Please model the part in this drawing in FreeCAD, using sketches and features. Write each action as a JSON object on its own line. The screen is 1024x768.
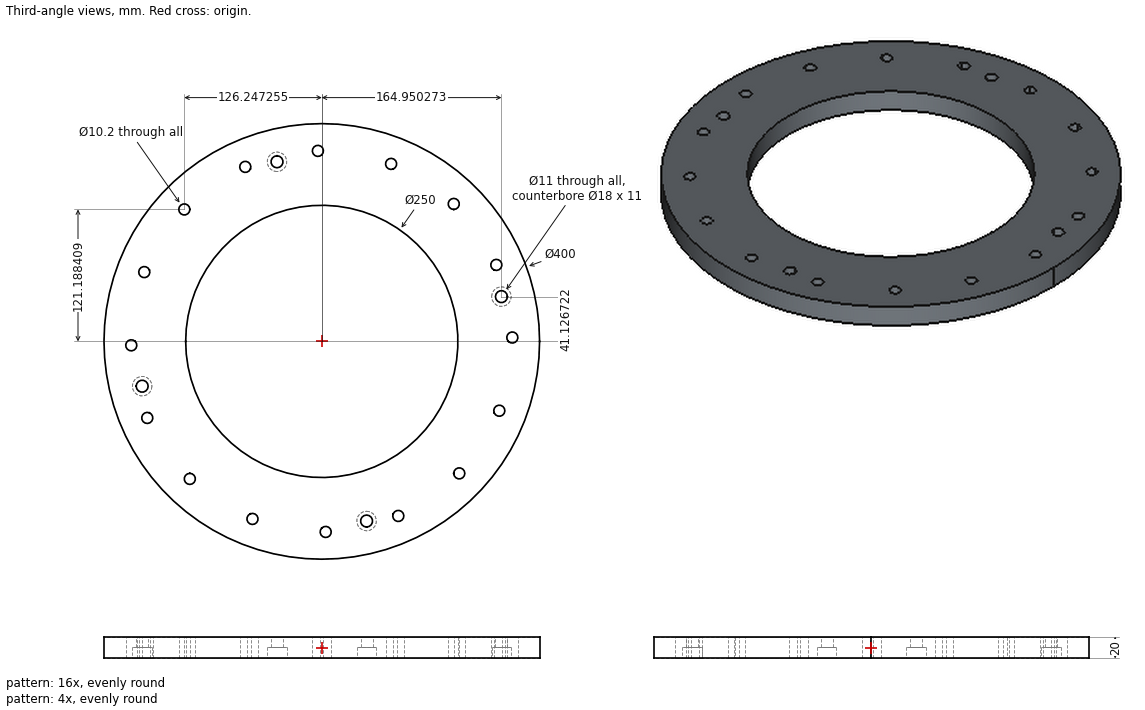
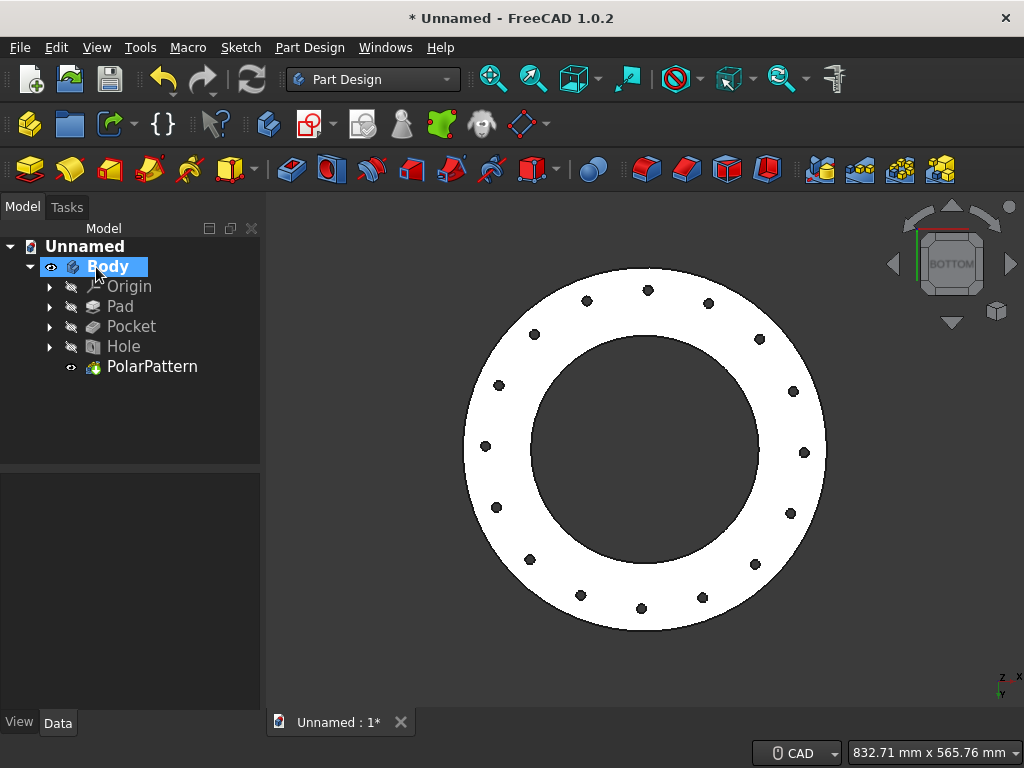
{"action": "left_click", "coordinate": [489, 396]}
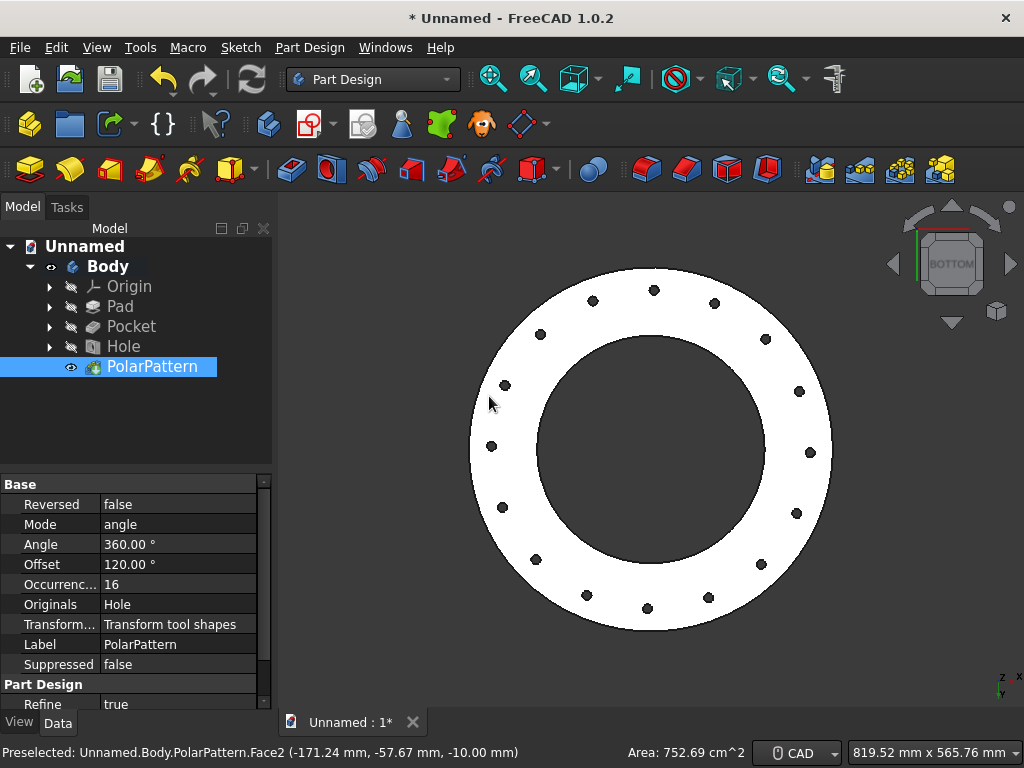
{"action": "left_click", "coordinate": [310, 124]}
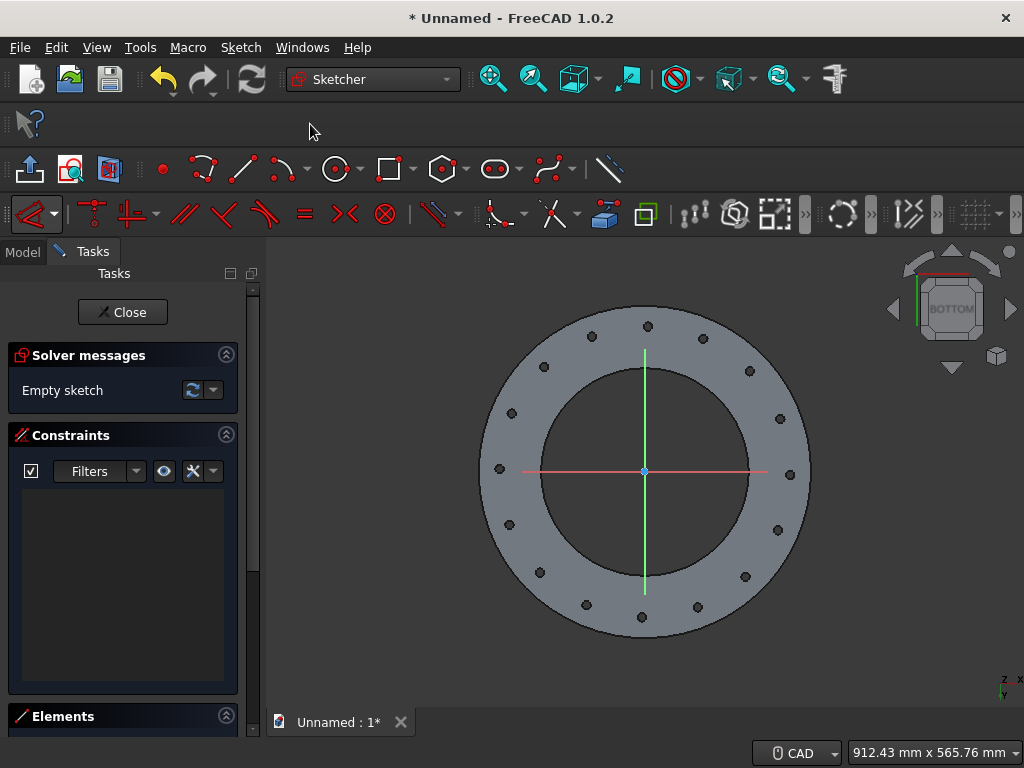
{"action": "scroll", "coordinate": [793, 508], "scroll_direction": "up", "scroll_amount": 15}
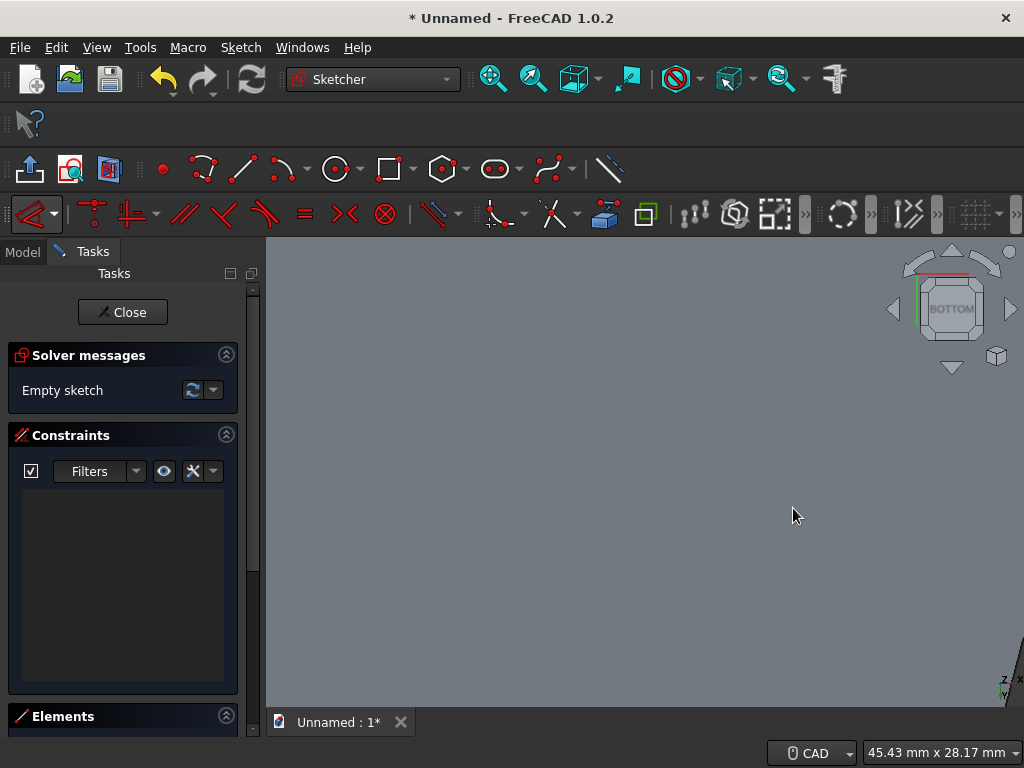
{"action": "scroll", "coordinate": [518, 436], "scroll_direction": "up", "scroll_amount": 2}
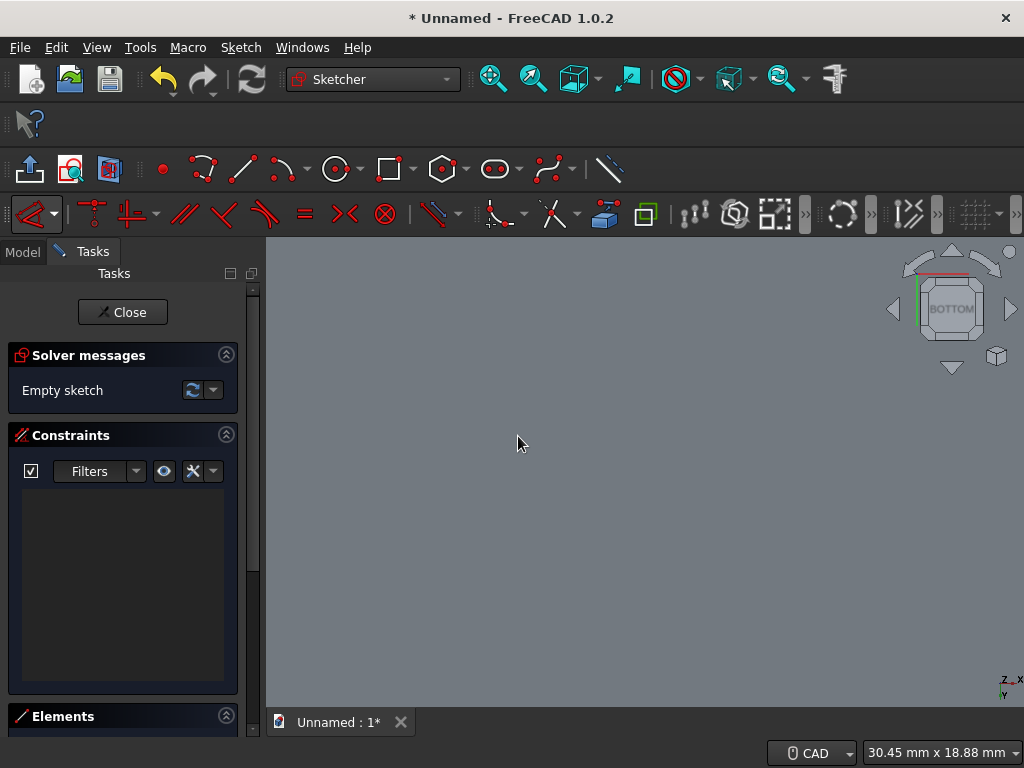
{"action": "left_click", "coordinate": [336, 170]}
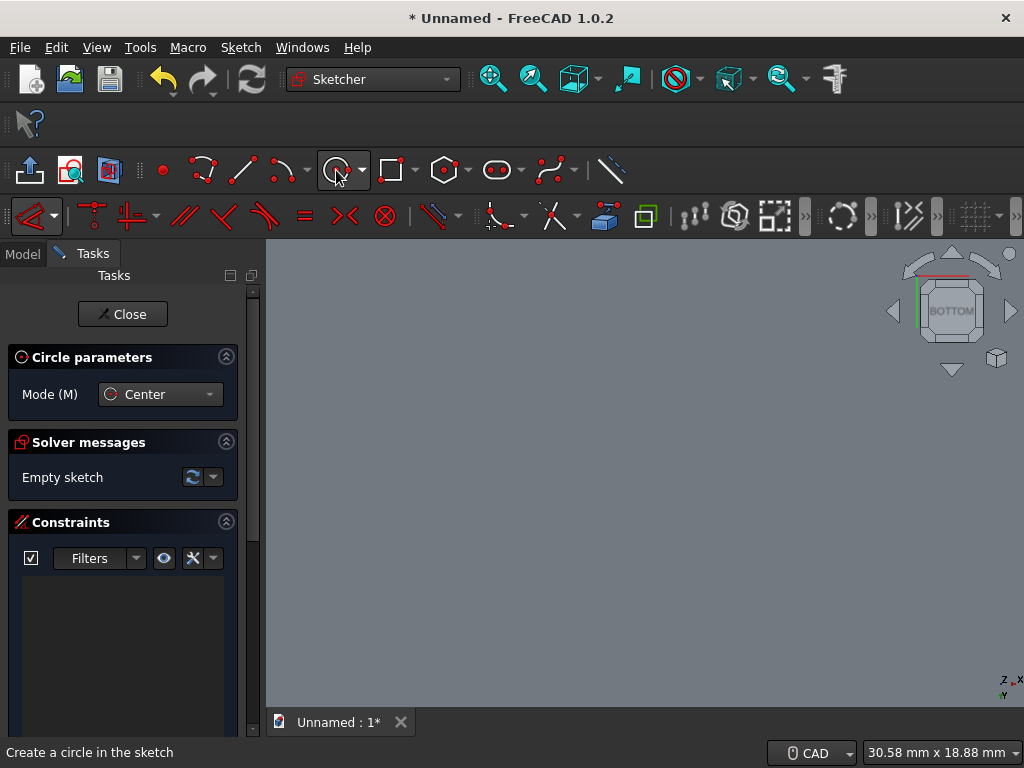
{"action": "left_click", "coordinate": [577, 473]}
{"action": "left_click", "coordinate": [673, 376]}
{"action": "key", "text": "Escape"}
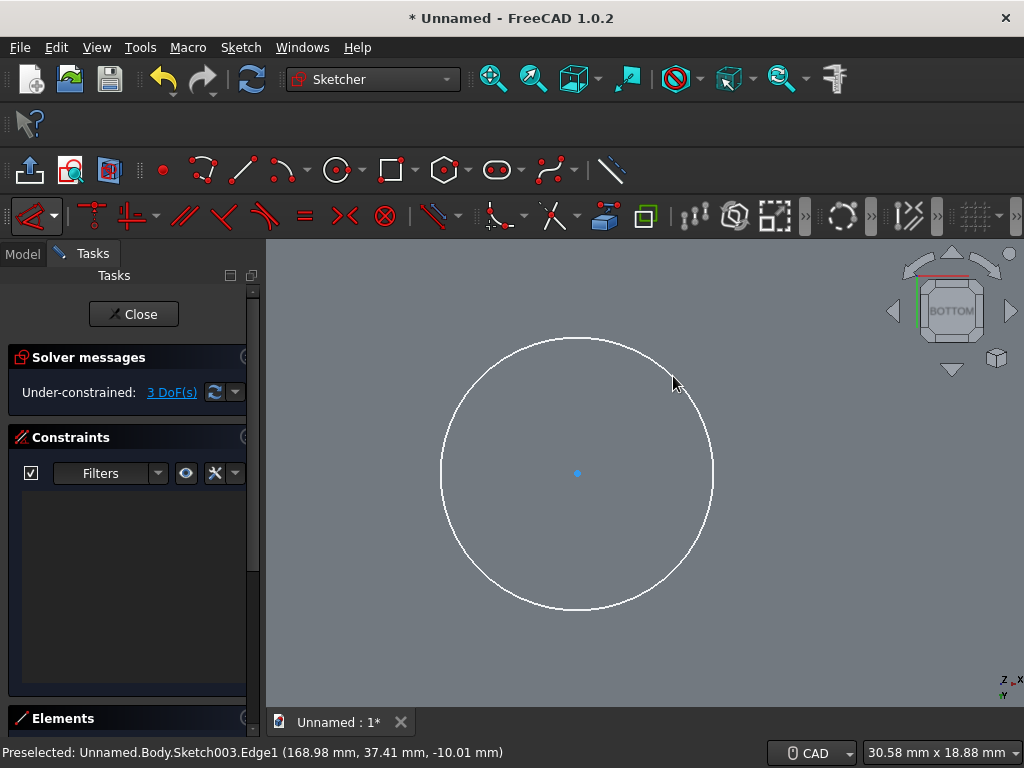
{"action": "left_click", "coordinate": [673, 377]}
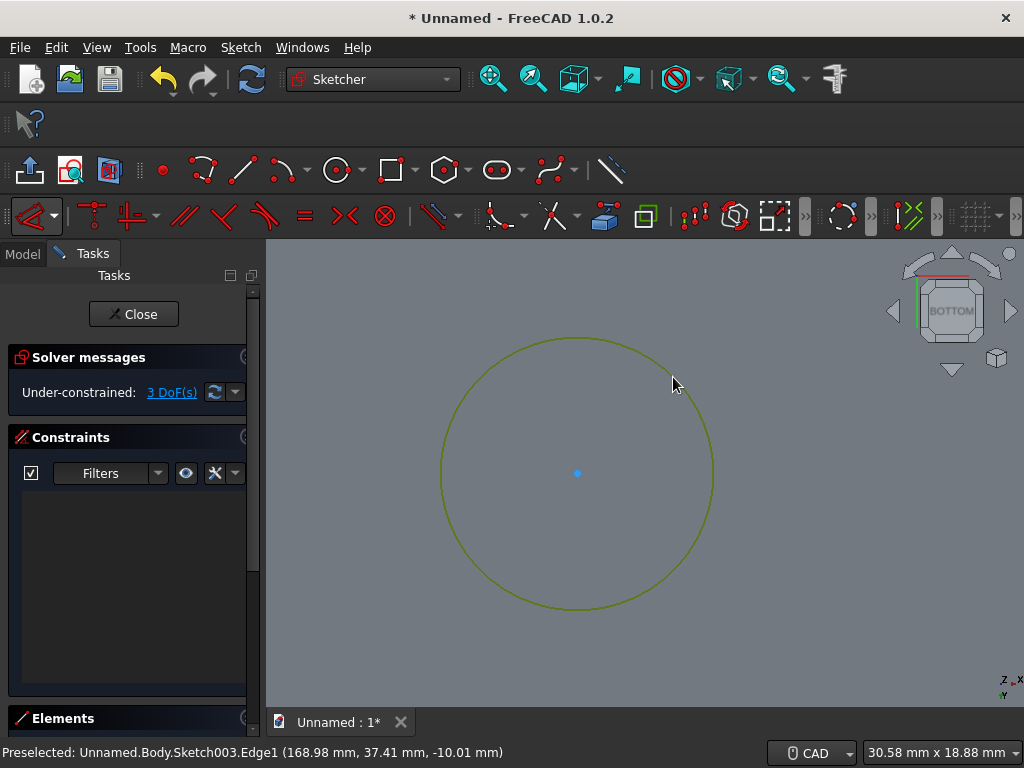
{"action": "left_click", "coordinate": [56, 216]}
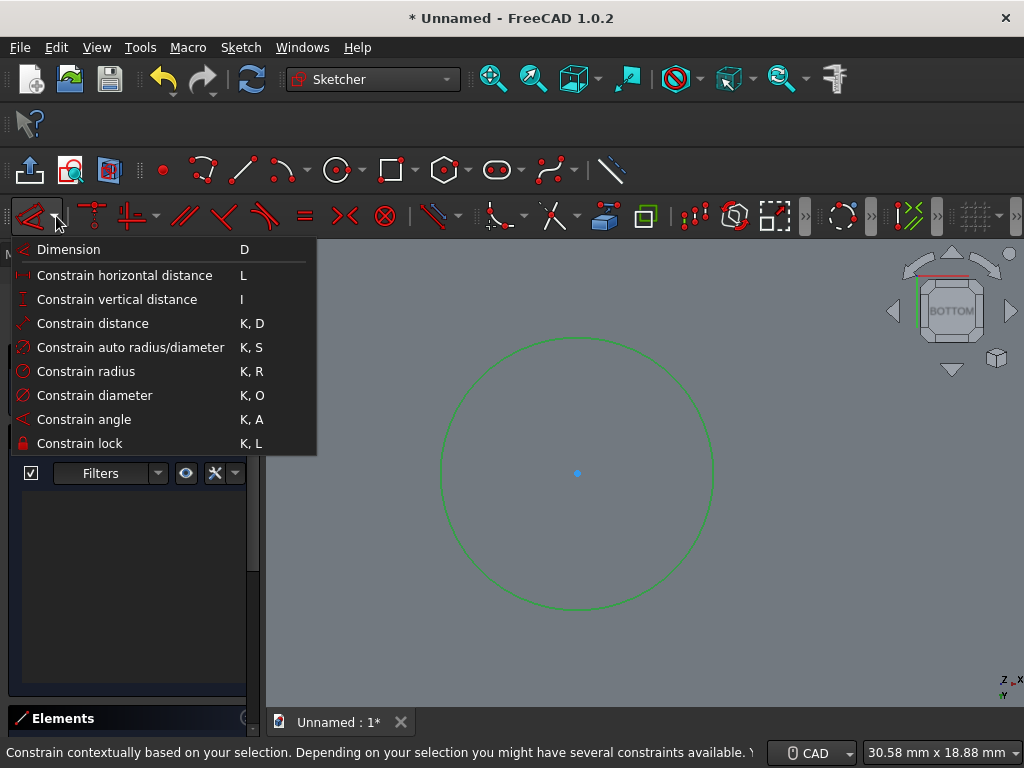
{"action": "left_click", "coordinate": [164, 395]}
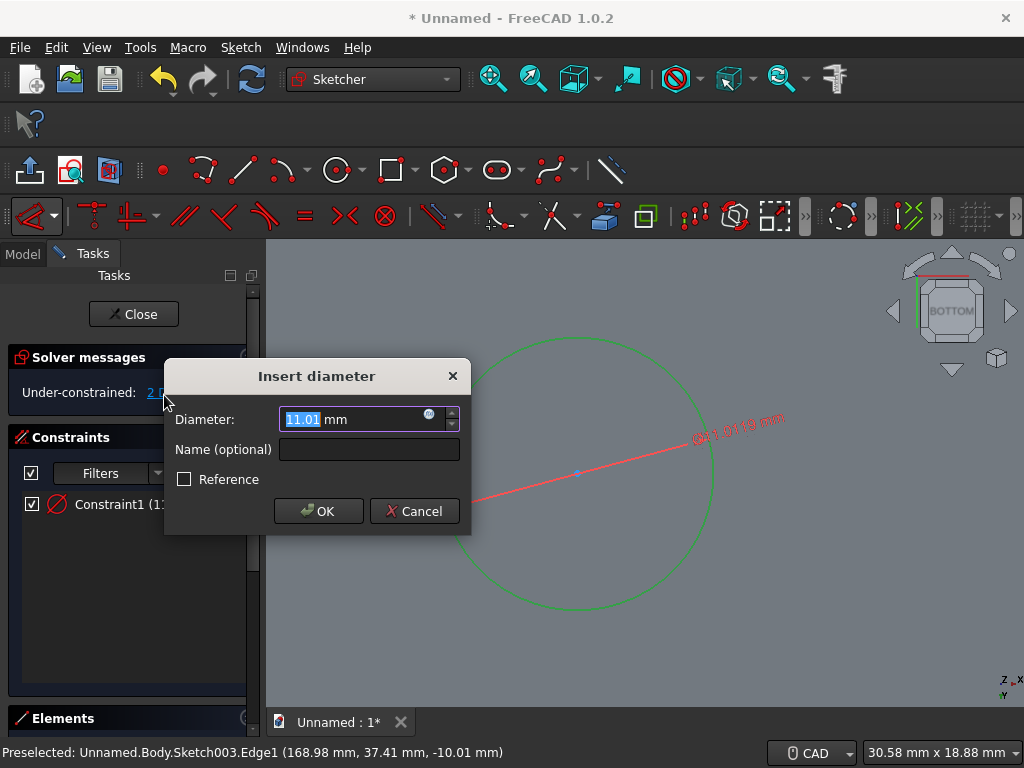
{"action": "type", "text": "11"}
{"action": "key", "text": "Return"}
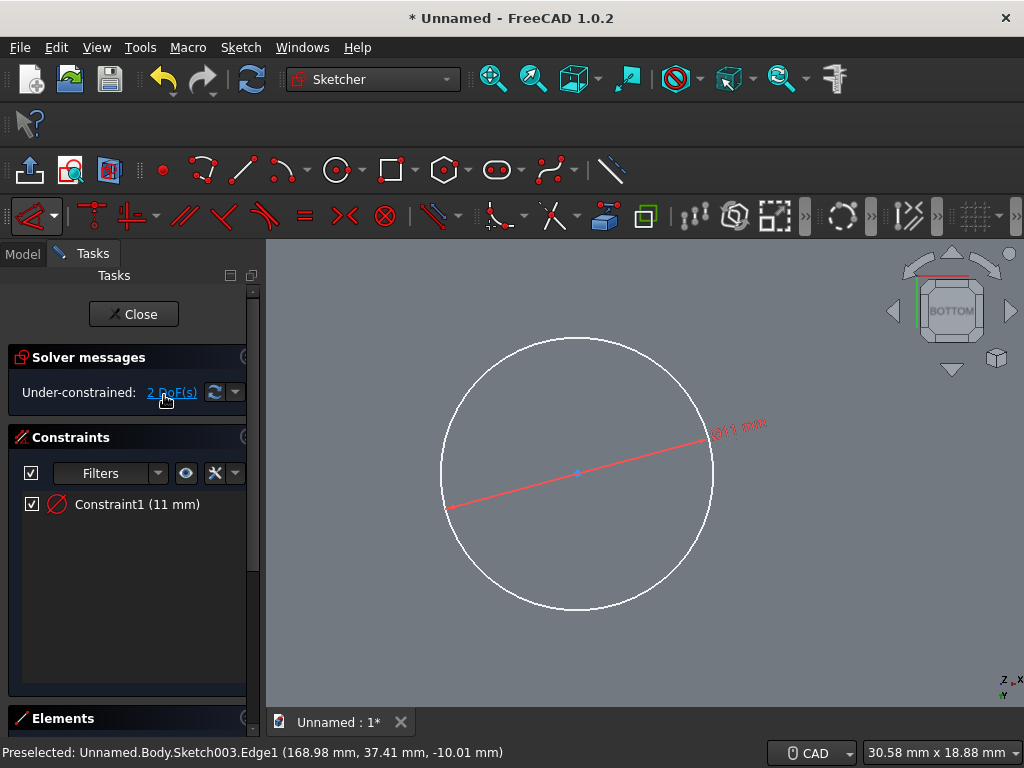
{"action": "left_click", "coordinate": [577, 474]}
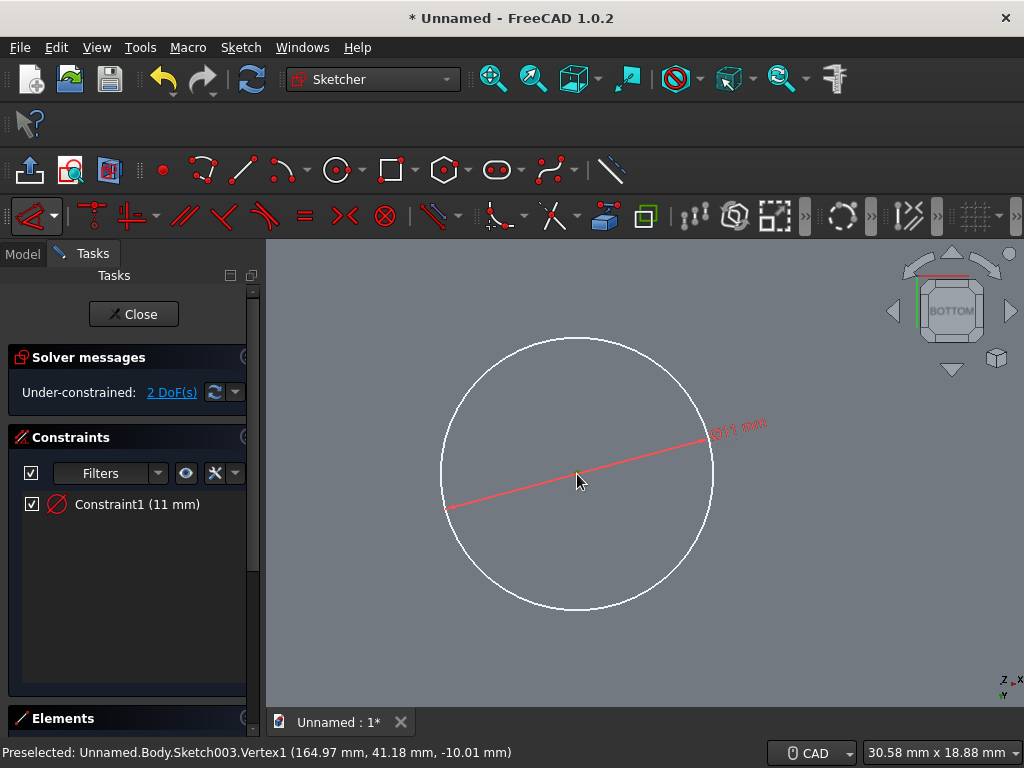
{"action": "left_click", "coordinate": [56, 216]}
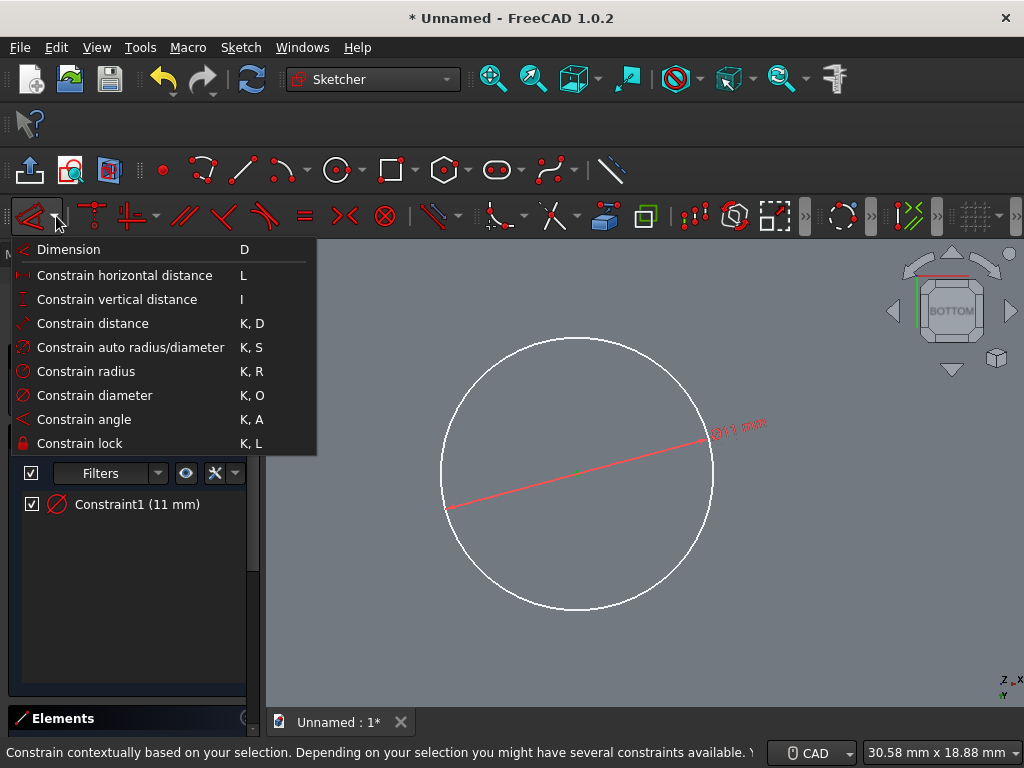
{"action": "left_click", "coordinate": [164, 299]}